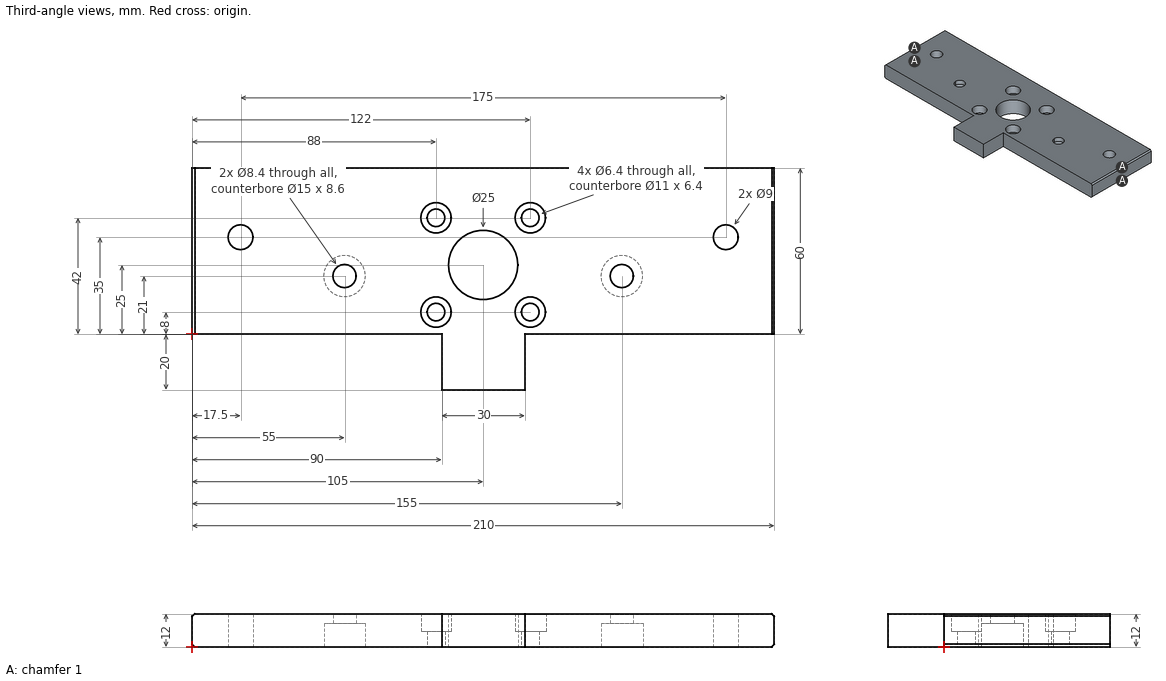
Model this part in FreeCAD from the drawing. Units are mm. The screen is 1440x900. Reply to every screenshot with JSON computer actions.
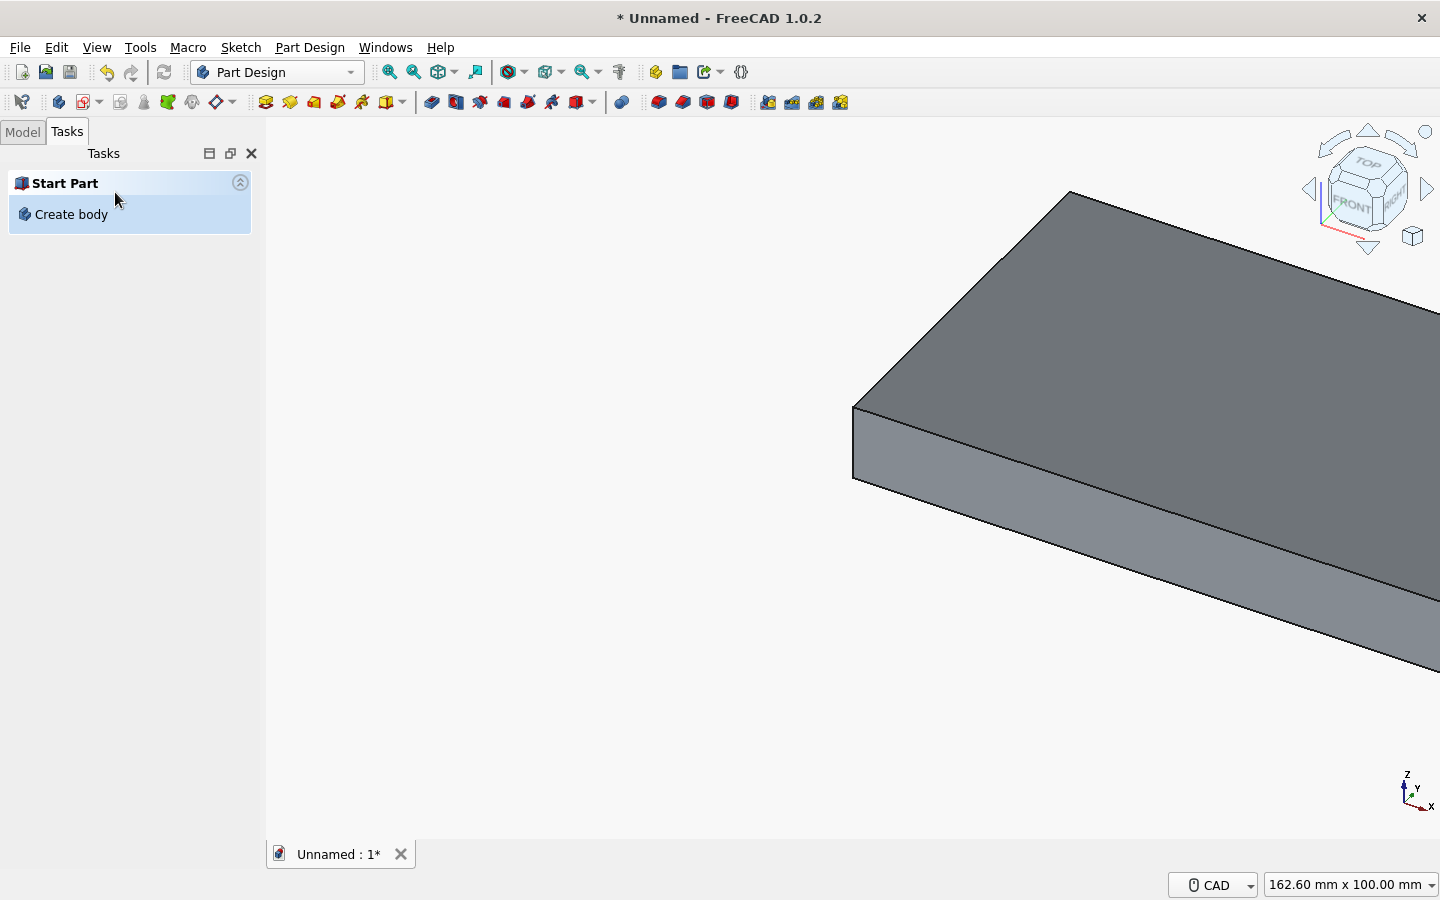
{"action": "left_click", "coordinate": [390, 72]}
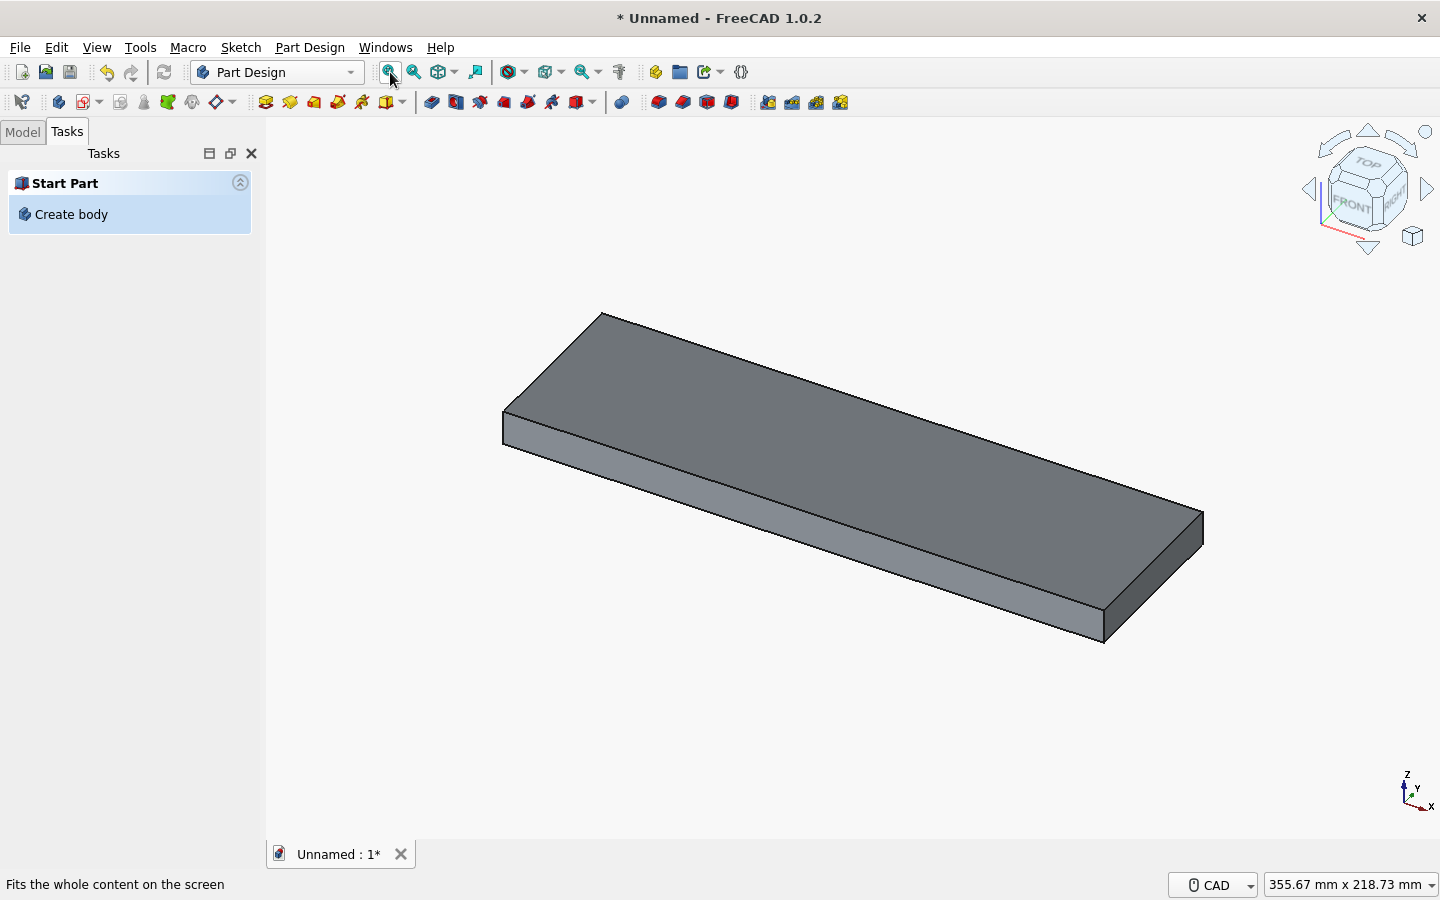
{"action": "left_click", "coordinate": [1025, 518]}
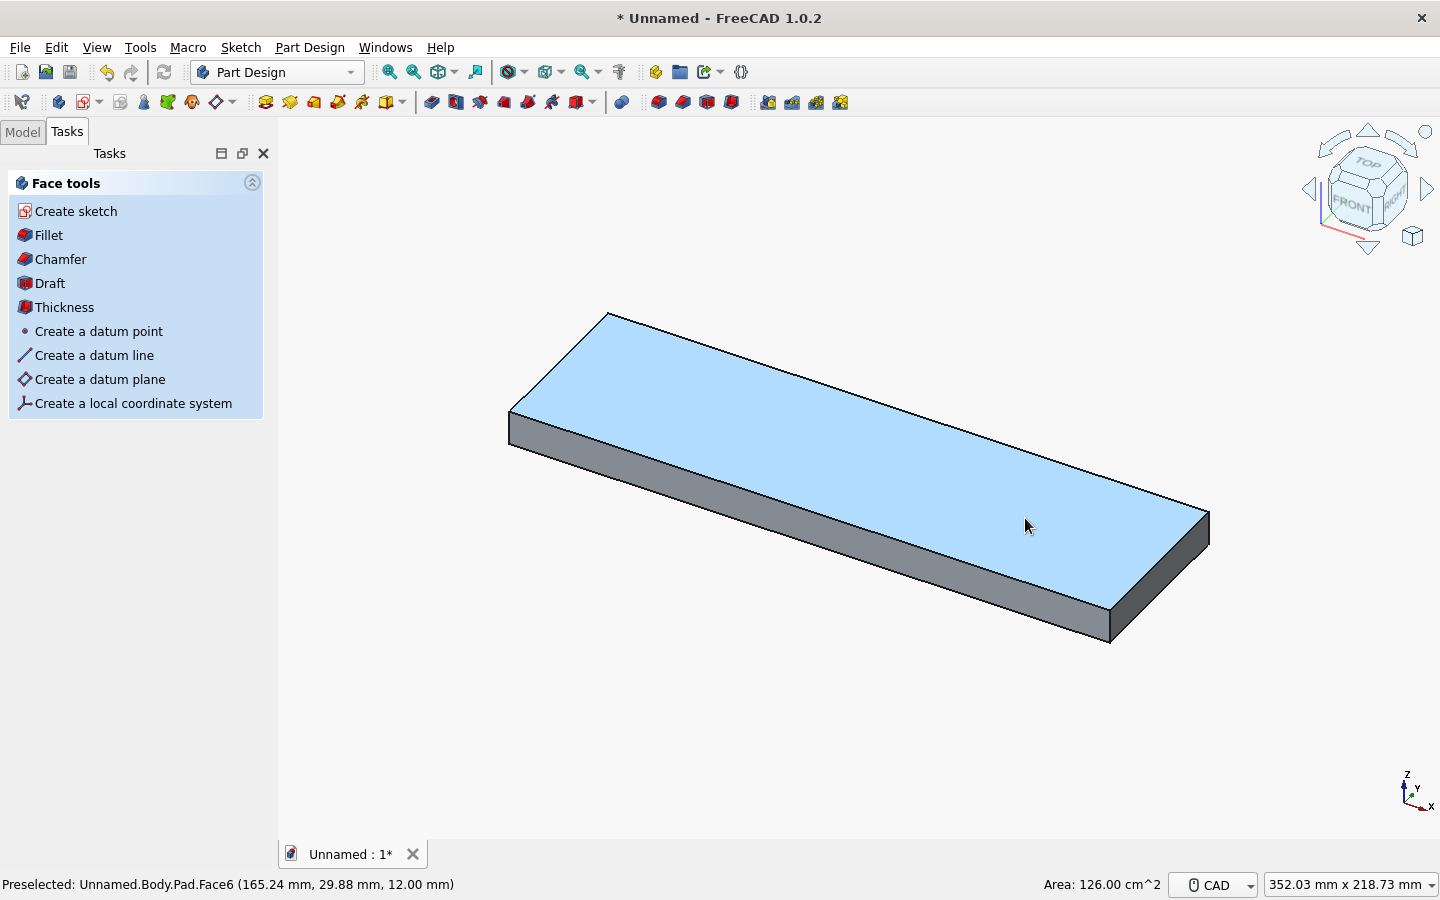
{"action": "left_click", "coordinate": [84, 102]}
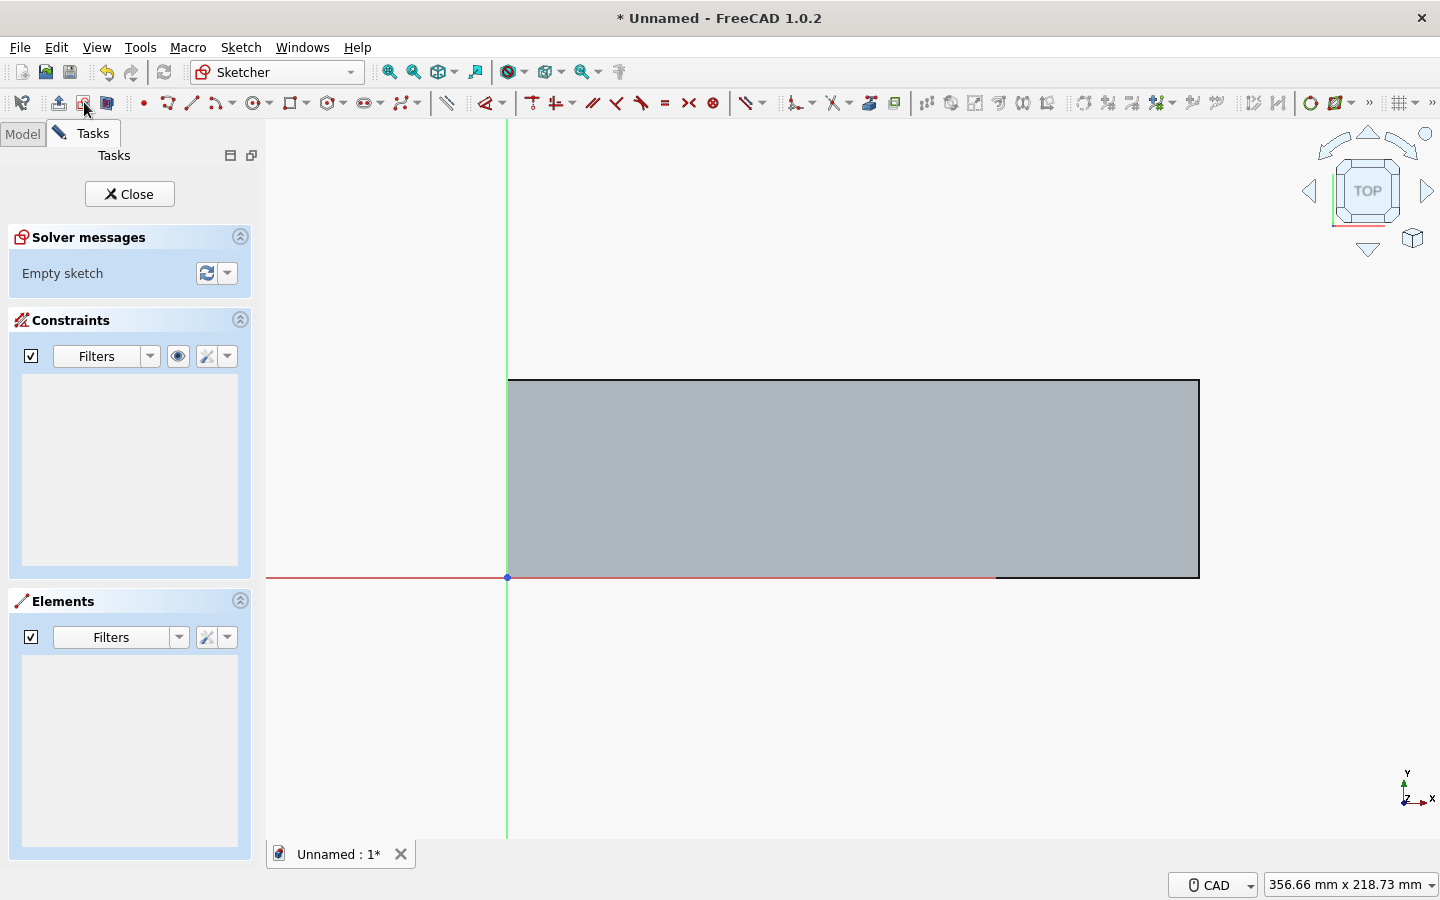
{"action": "scroll", "coordinate": [867, 499], "scroll_direction": "up", "scroll_amount": 9}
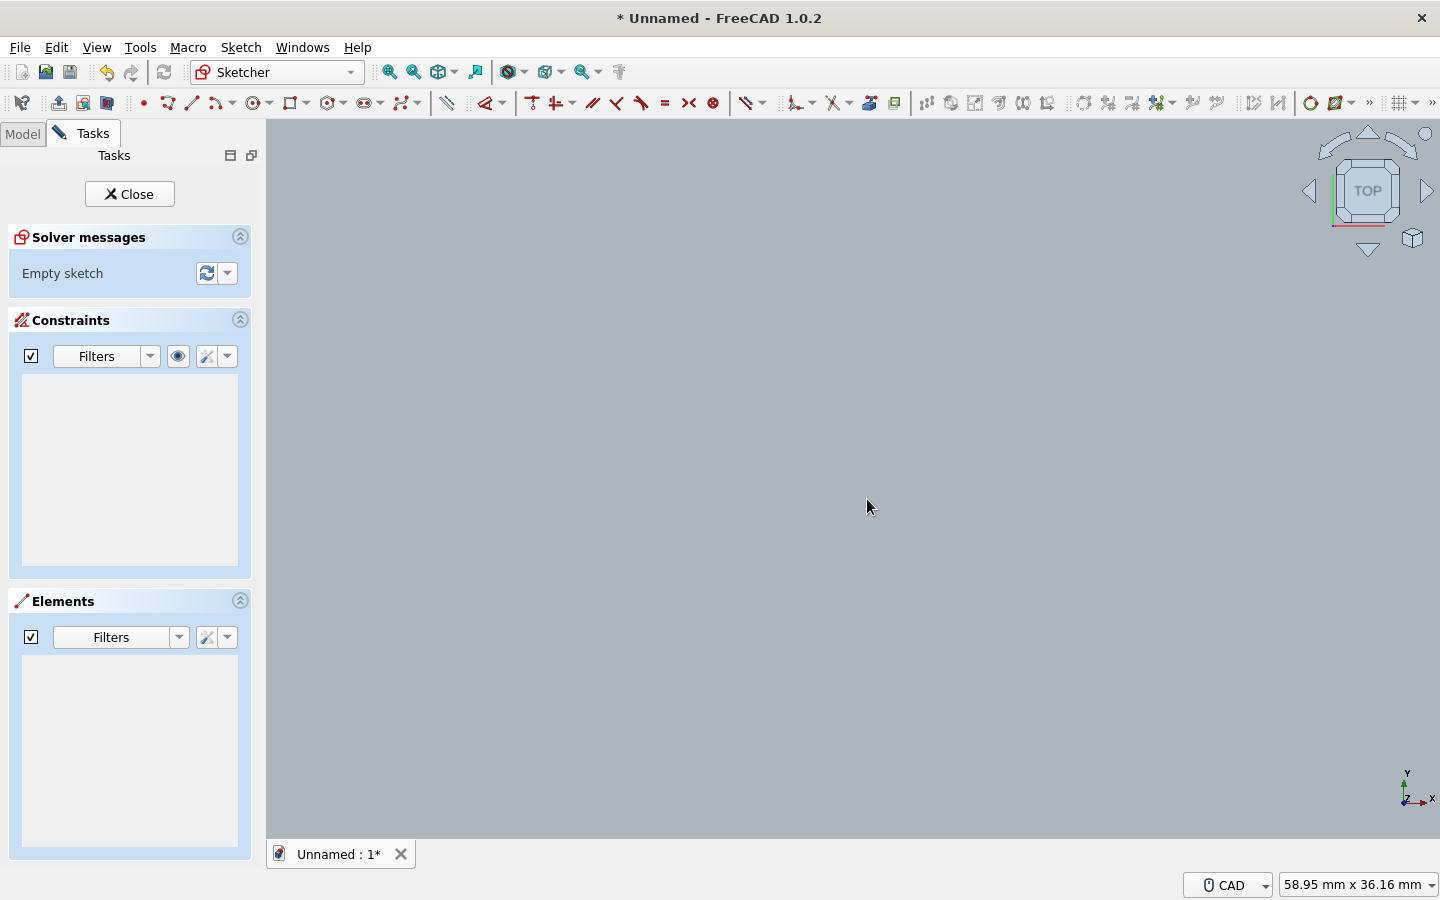
{"action": "key", "text": "g c"}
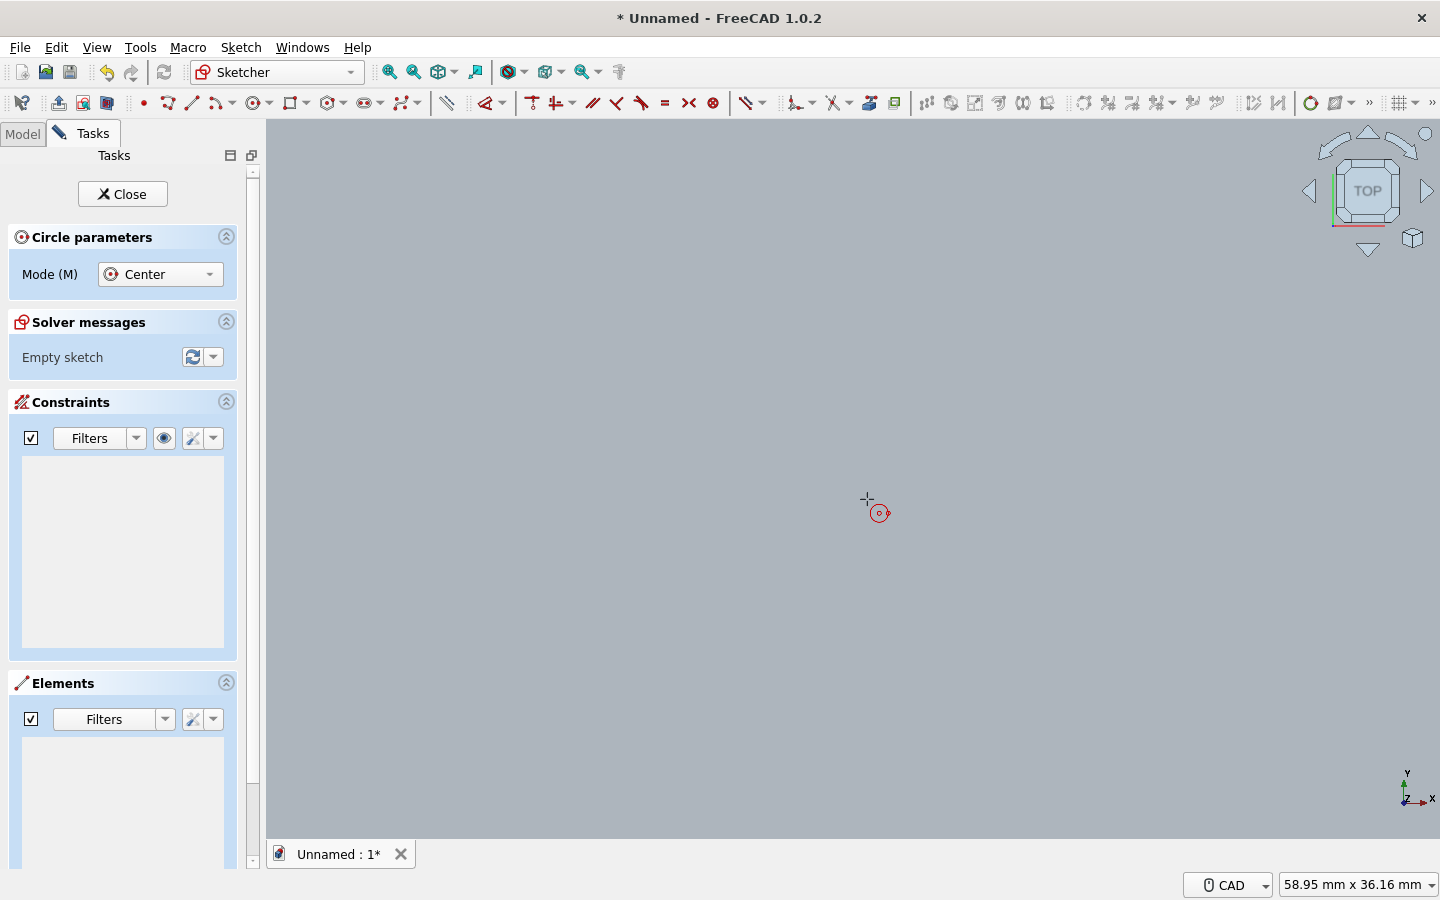
{"action": "left_click", "coordinate": [780, 475]}
{"action": "left_click", "coordinate": [956, 299]}
{"action": "key", "text": "Escape"}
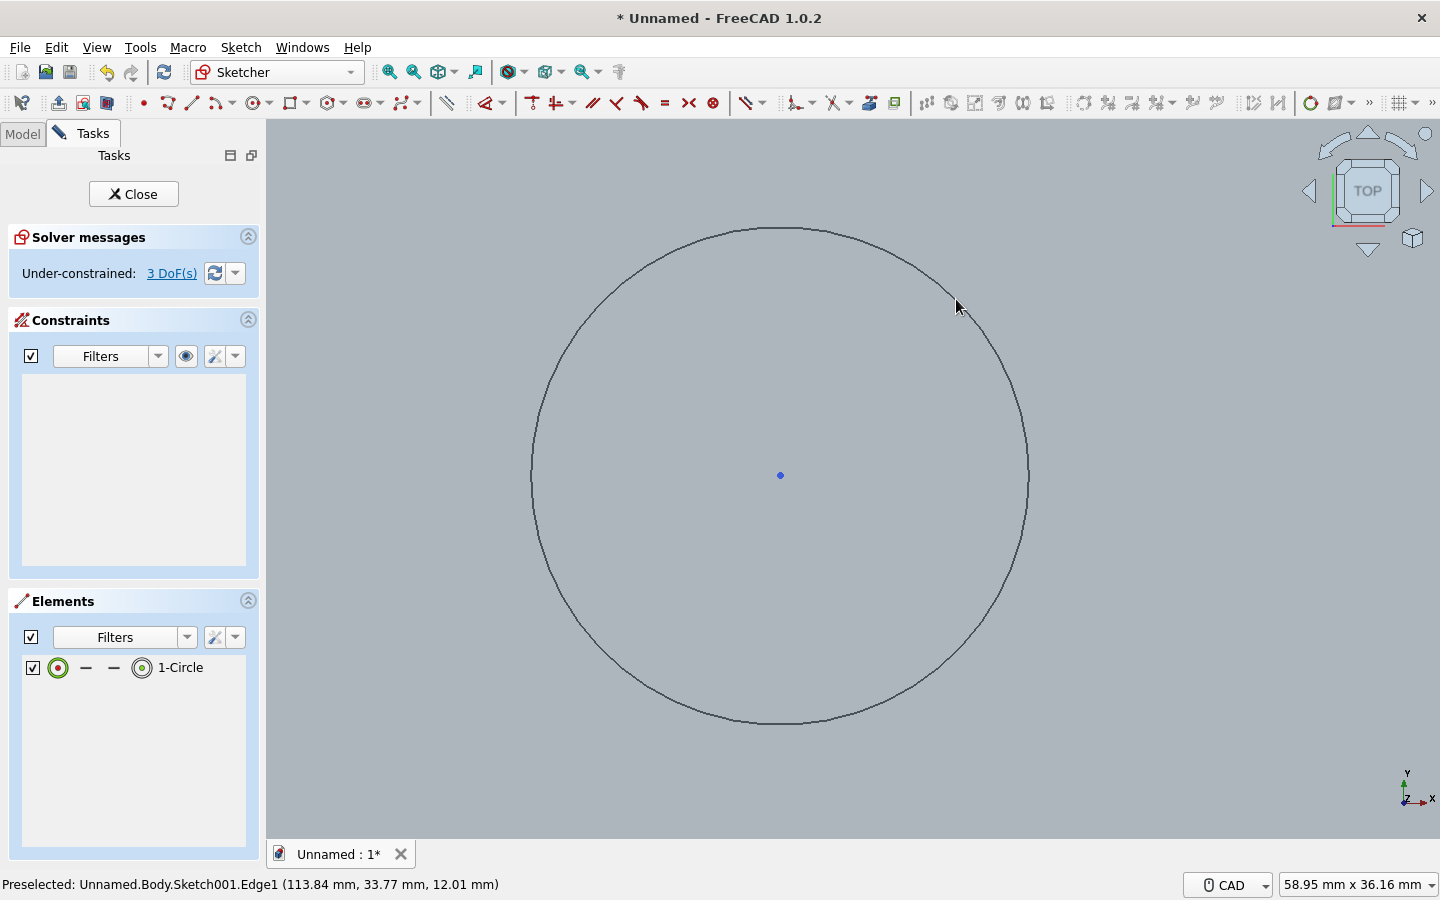
{"action": "key", "text": "d"}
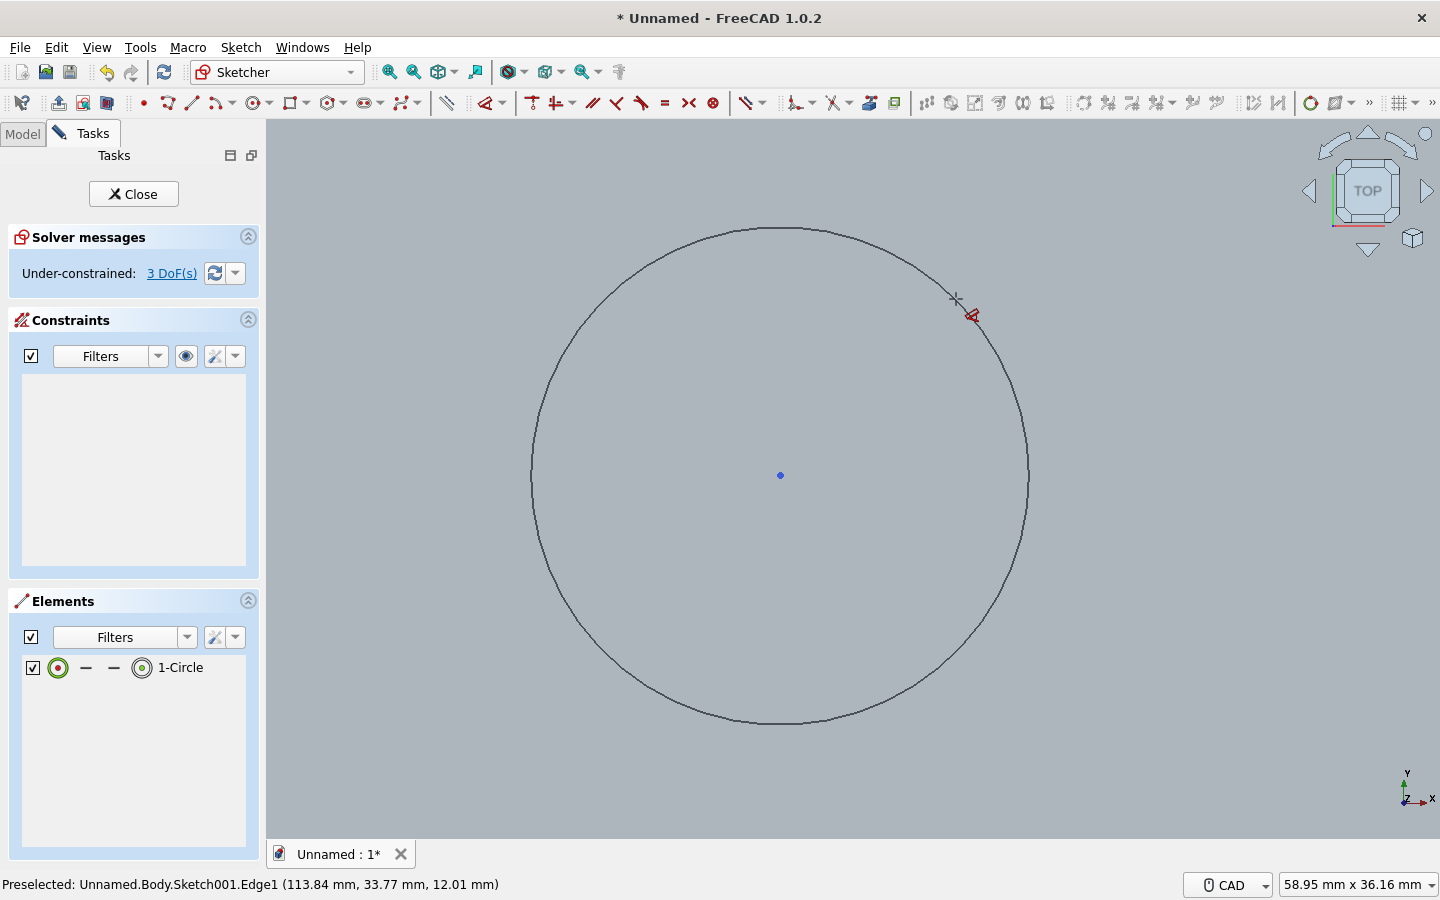
{"action": "left_click", "coordinate": [955, 299]}
{"action": "left_click", "coordinate": [977, 276]}